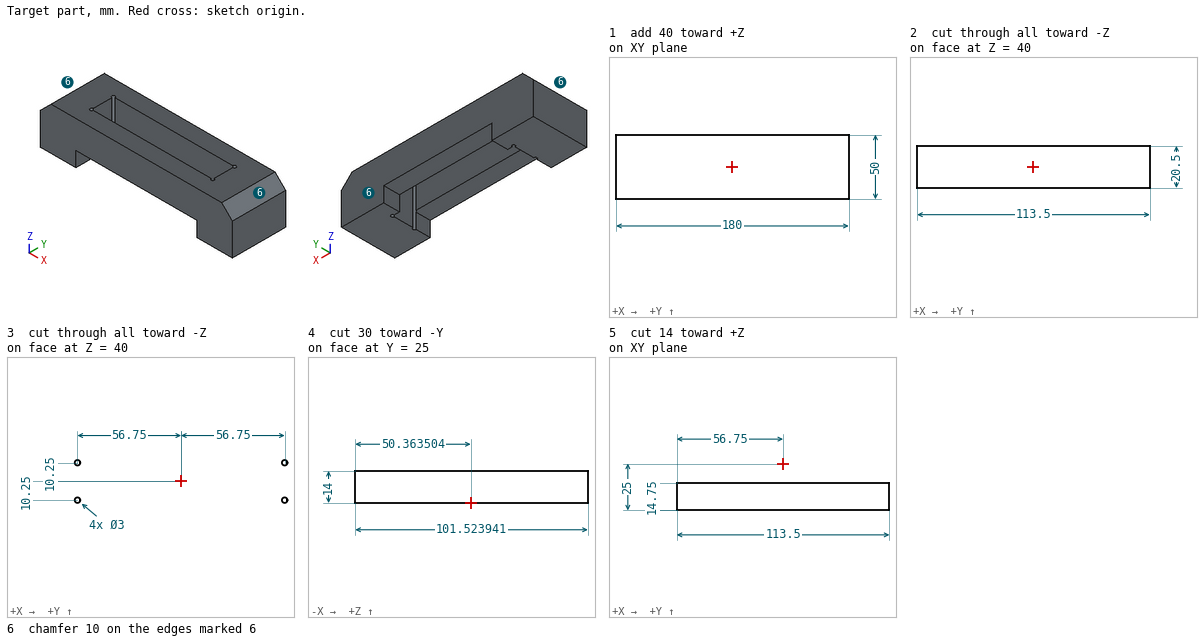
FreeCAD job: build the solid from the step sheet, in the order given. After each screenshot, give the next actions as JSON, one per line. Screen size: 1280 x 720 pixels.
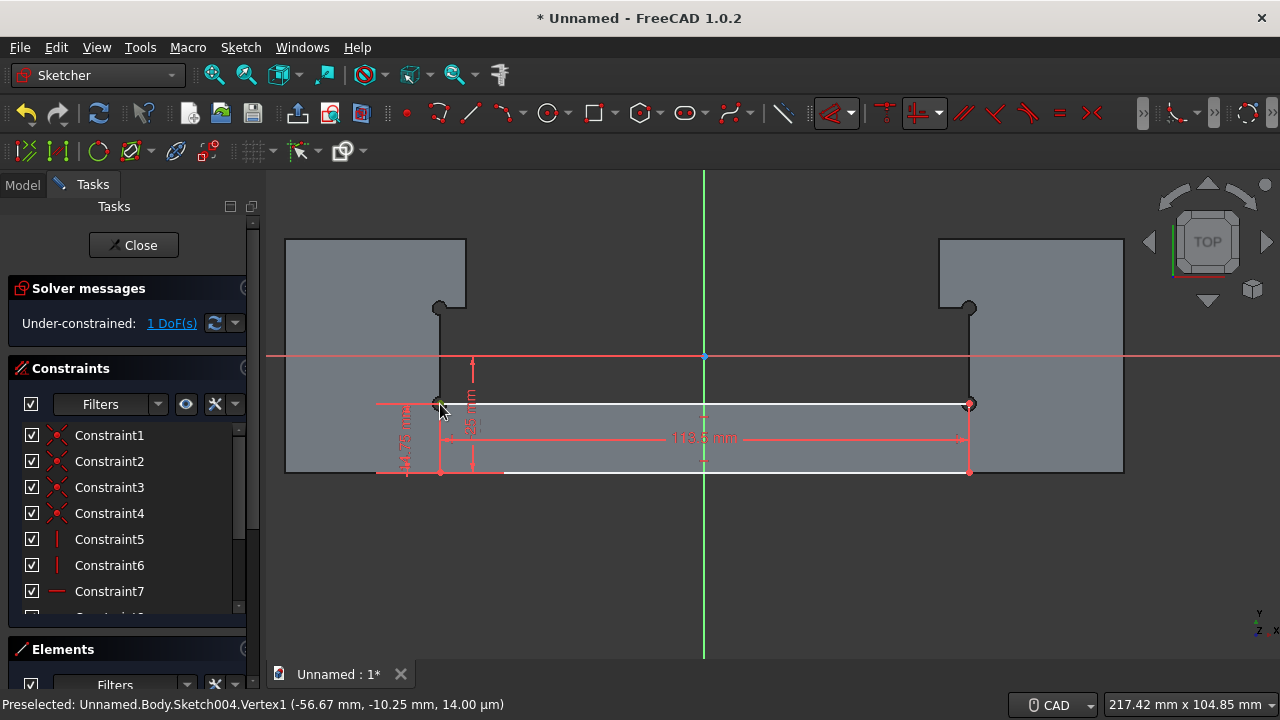
{"action": "left_click", "coordinate": [854, 114]}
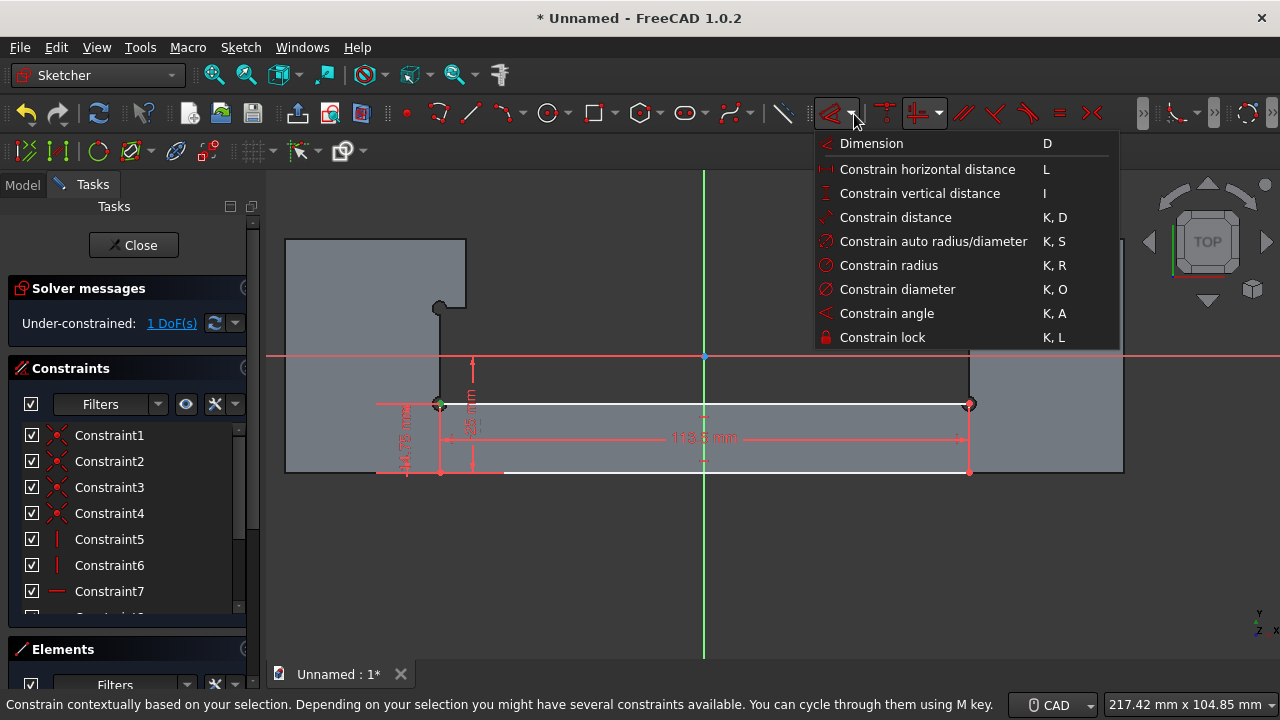
{"action": "left_click", "coordinate": [967, 169]}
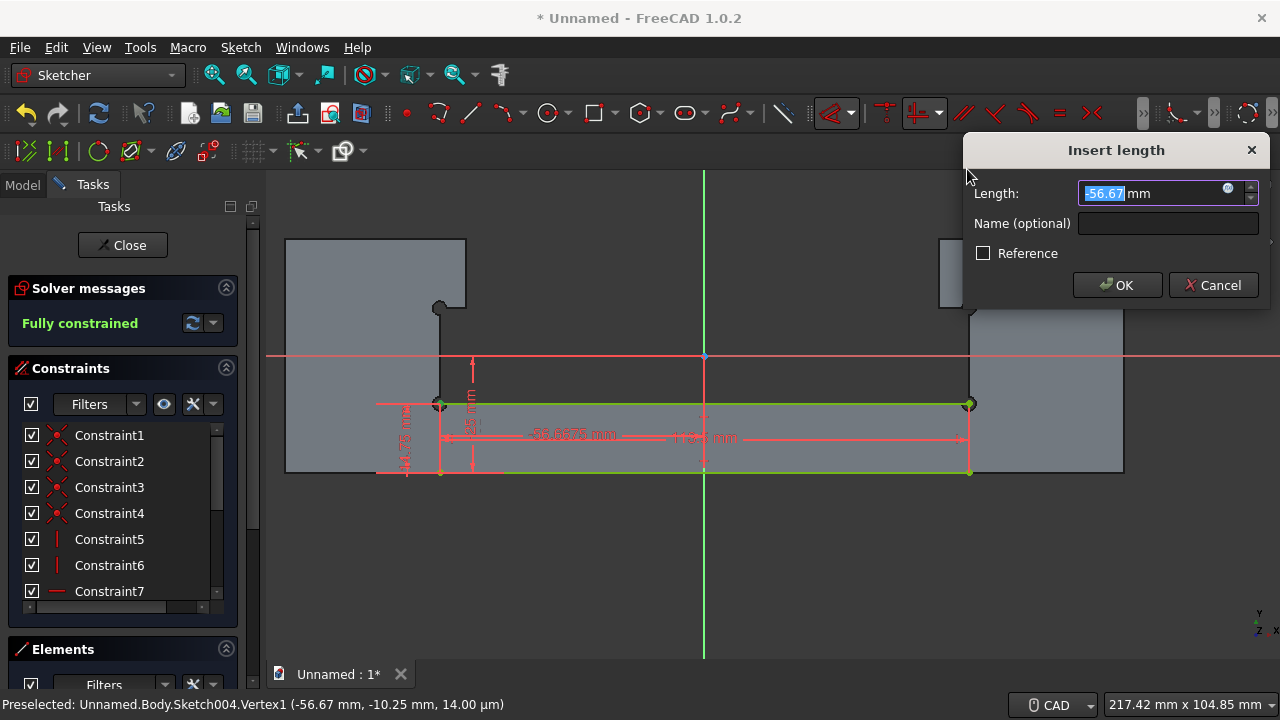
{"action": "type", "text": "-56.75"}
{"action": "key", "text": "Return"}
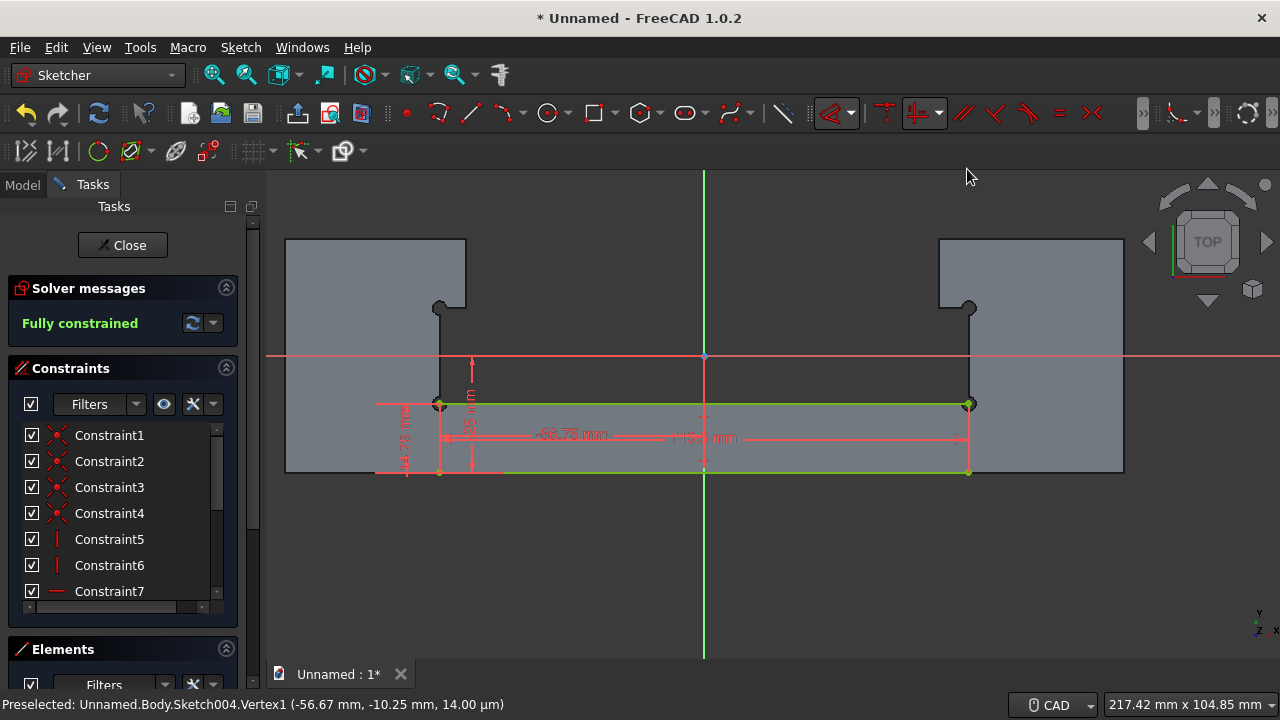
{"action": "left_click", "coordinate": [123, 245]}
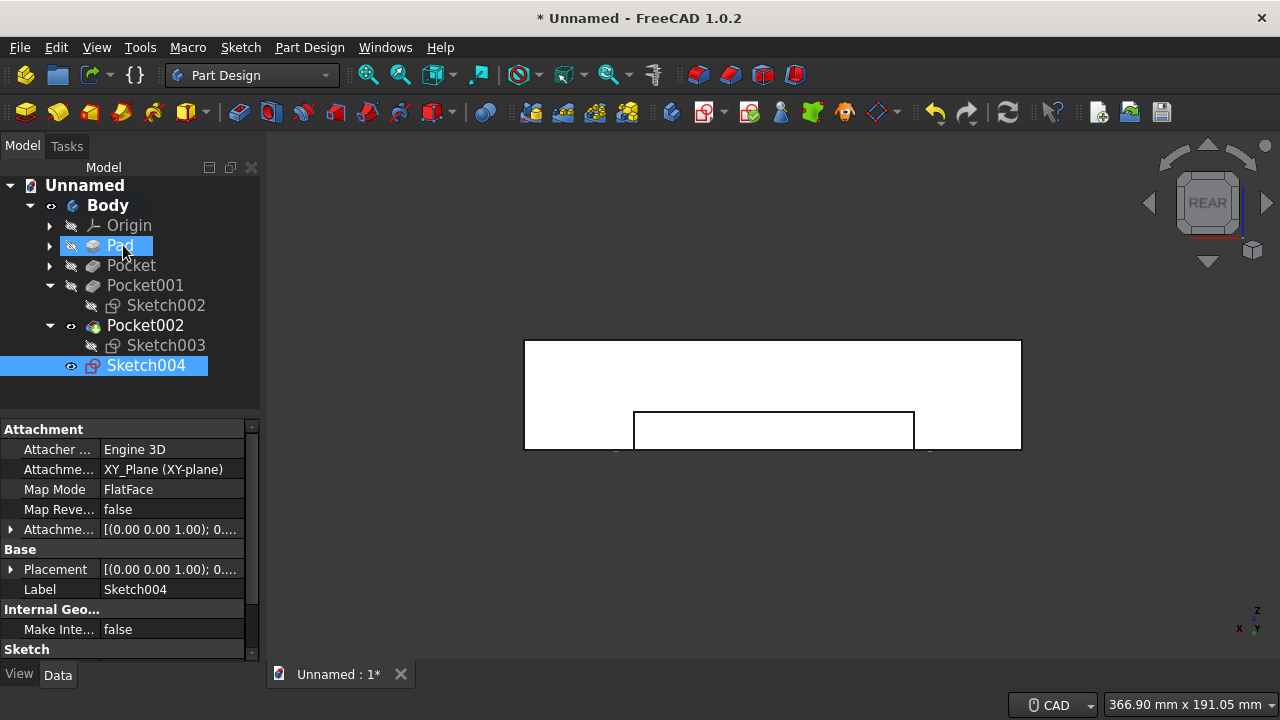
{"action": "left_click", "coordinate": [240, 112]}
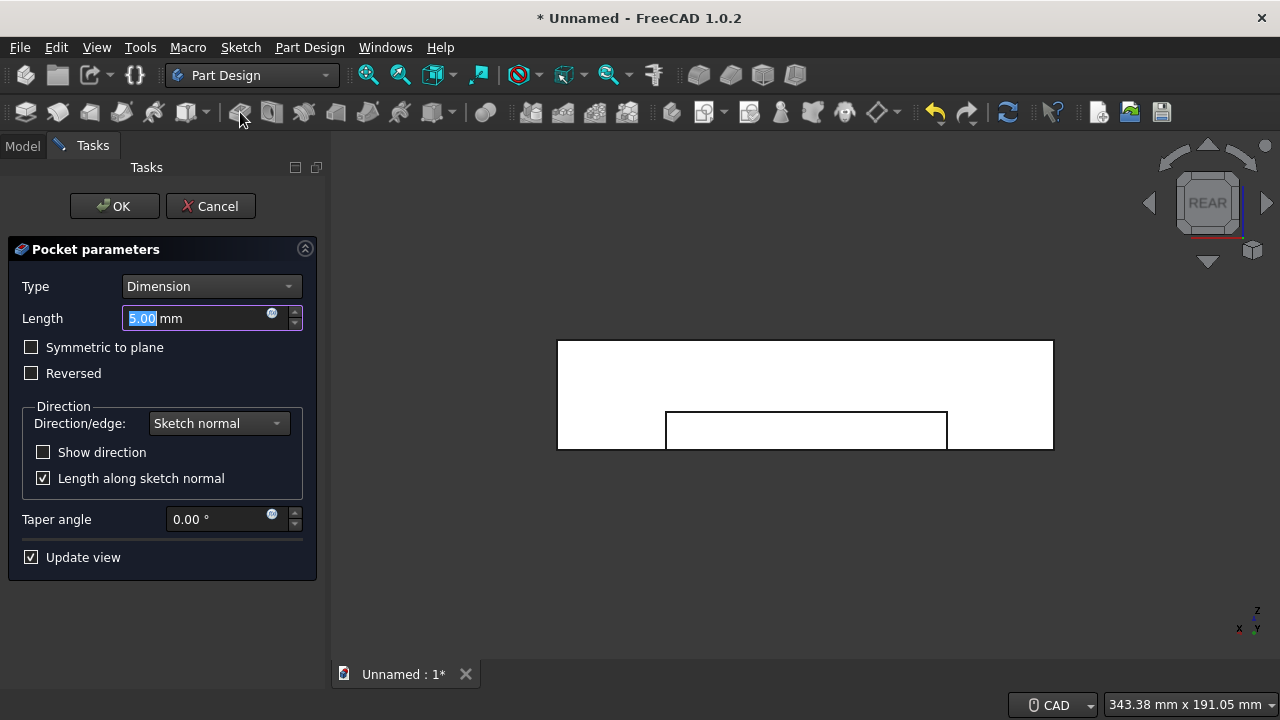
{"action": "type", "text": "14"}
{"action": "key", "text": "Tab"}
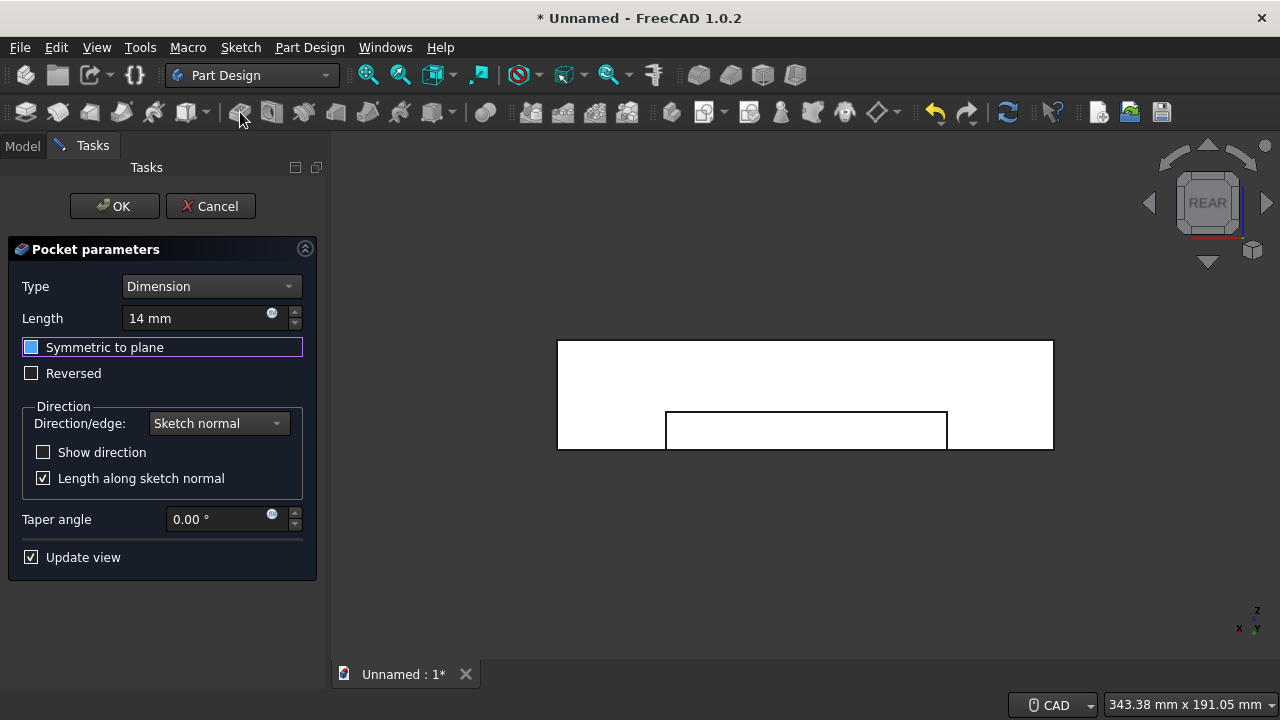
{"action": "left_click", "coordinate": [30, 373]}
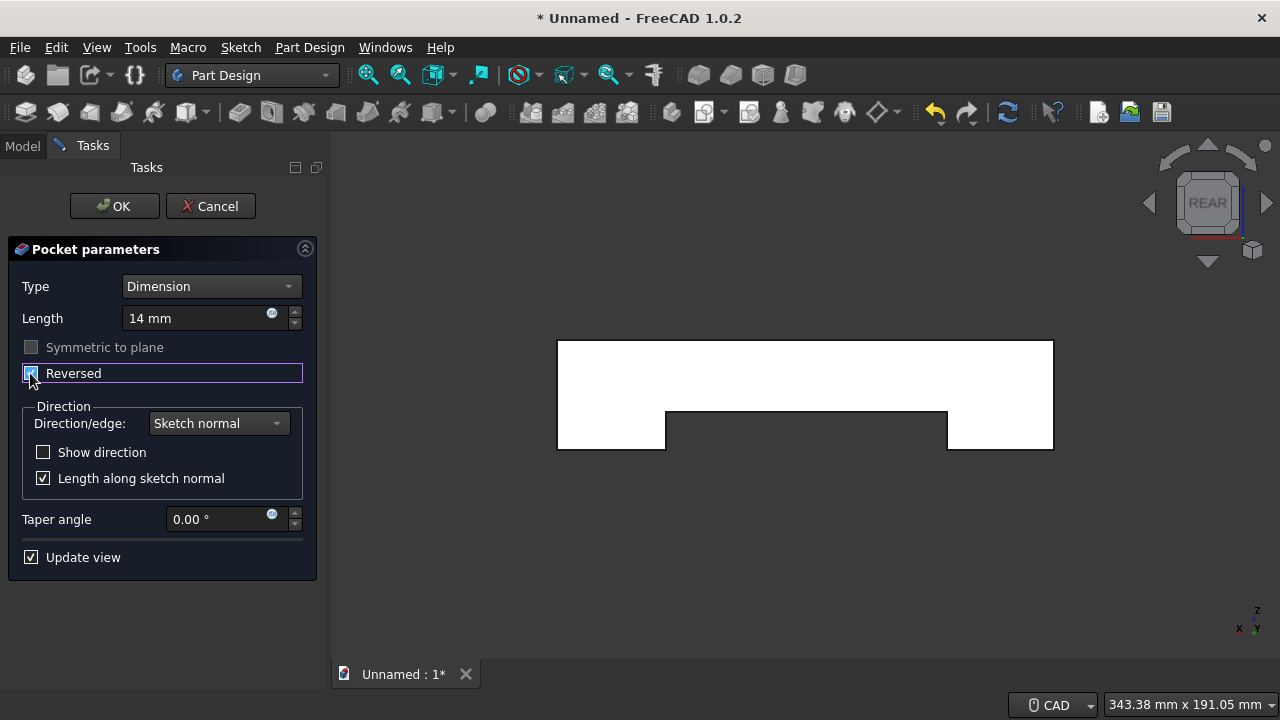
{"action": "left_click", "coordinate": [115, 206]}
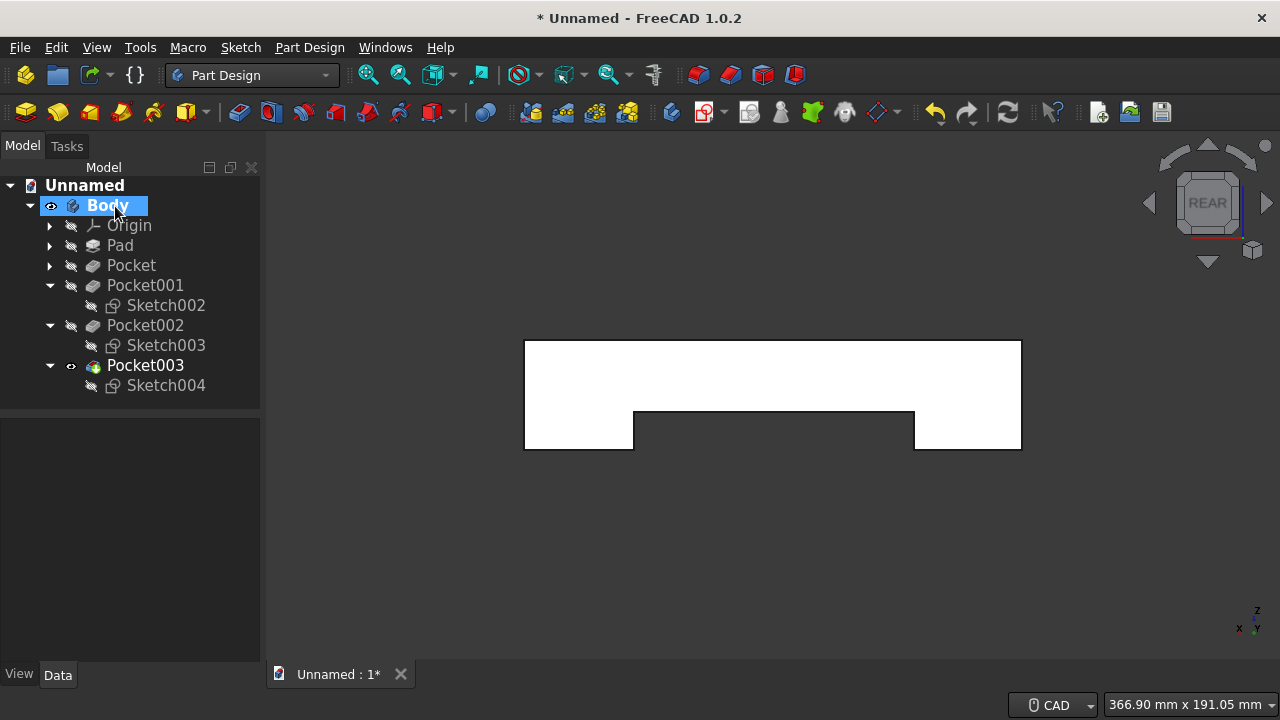
{"action": "key", "text": "0"}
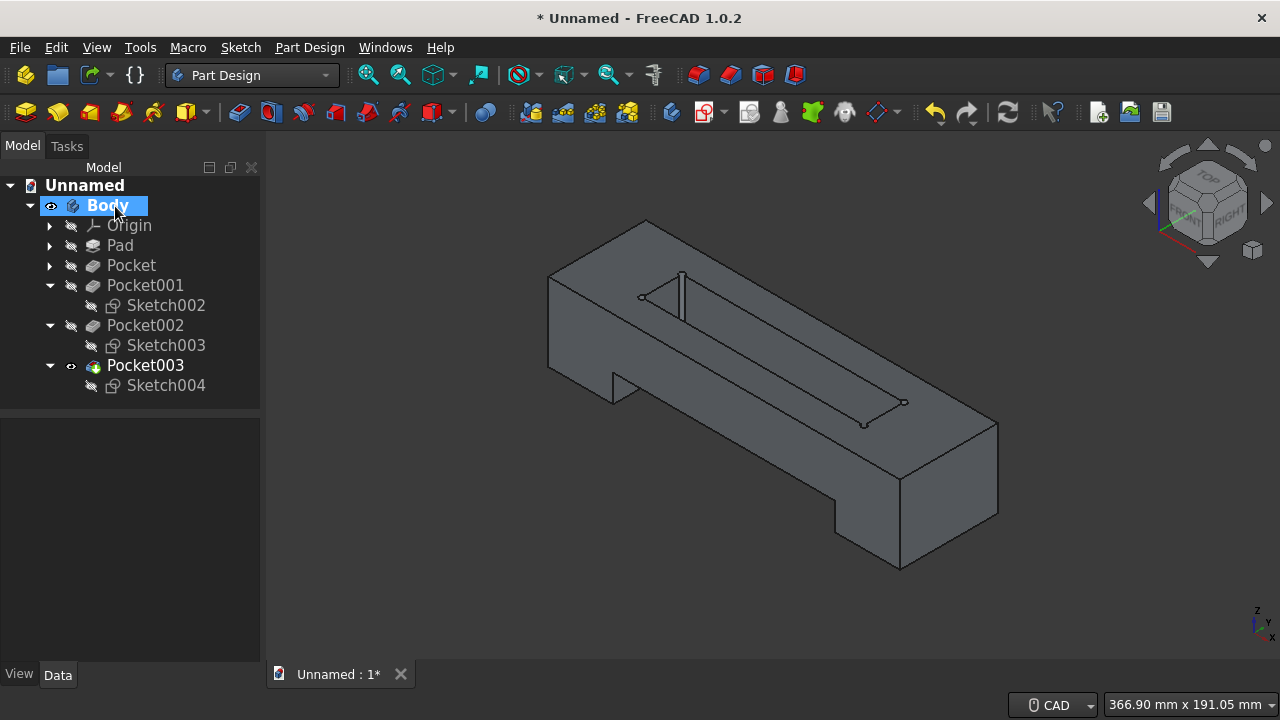
{"action": "left_click", "coordinate": [949, 450]}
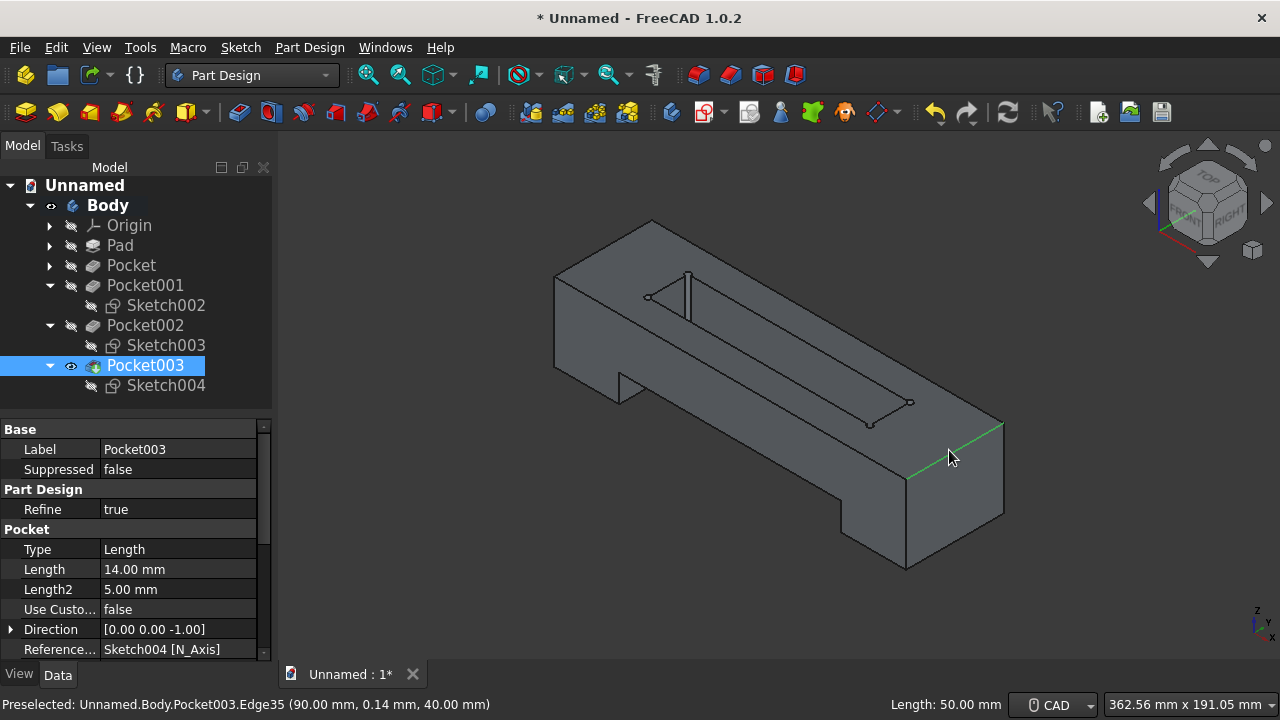
{"action": "key", "text": "2"}